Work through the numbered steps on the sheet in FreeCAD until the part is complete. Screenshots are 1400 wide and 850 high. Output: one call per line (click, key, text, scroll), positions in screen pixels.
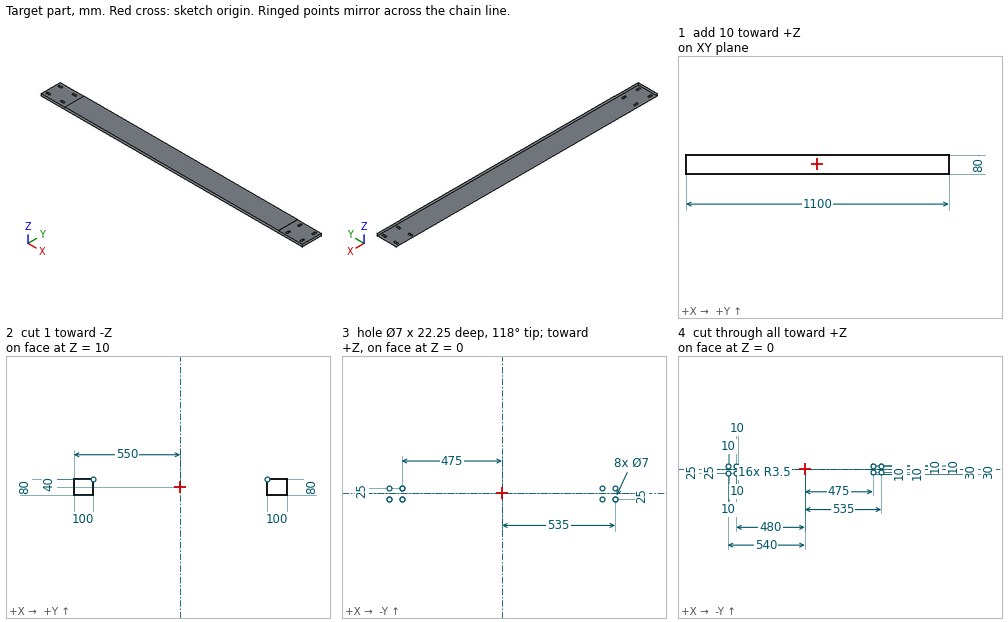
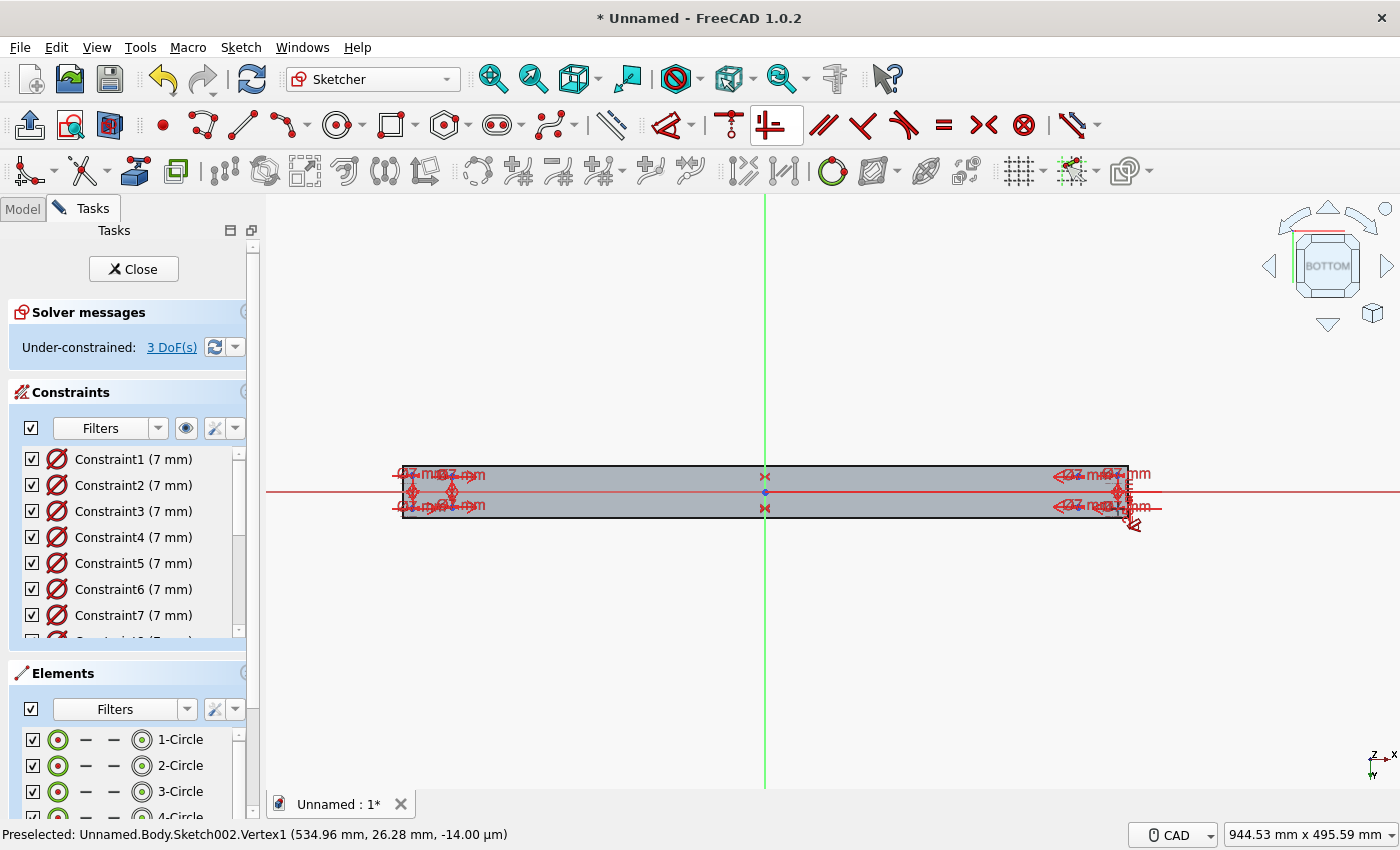
scroll(452, 477, up, 5)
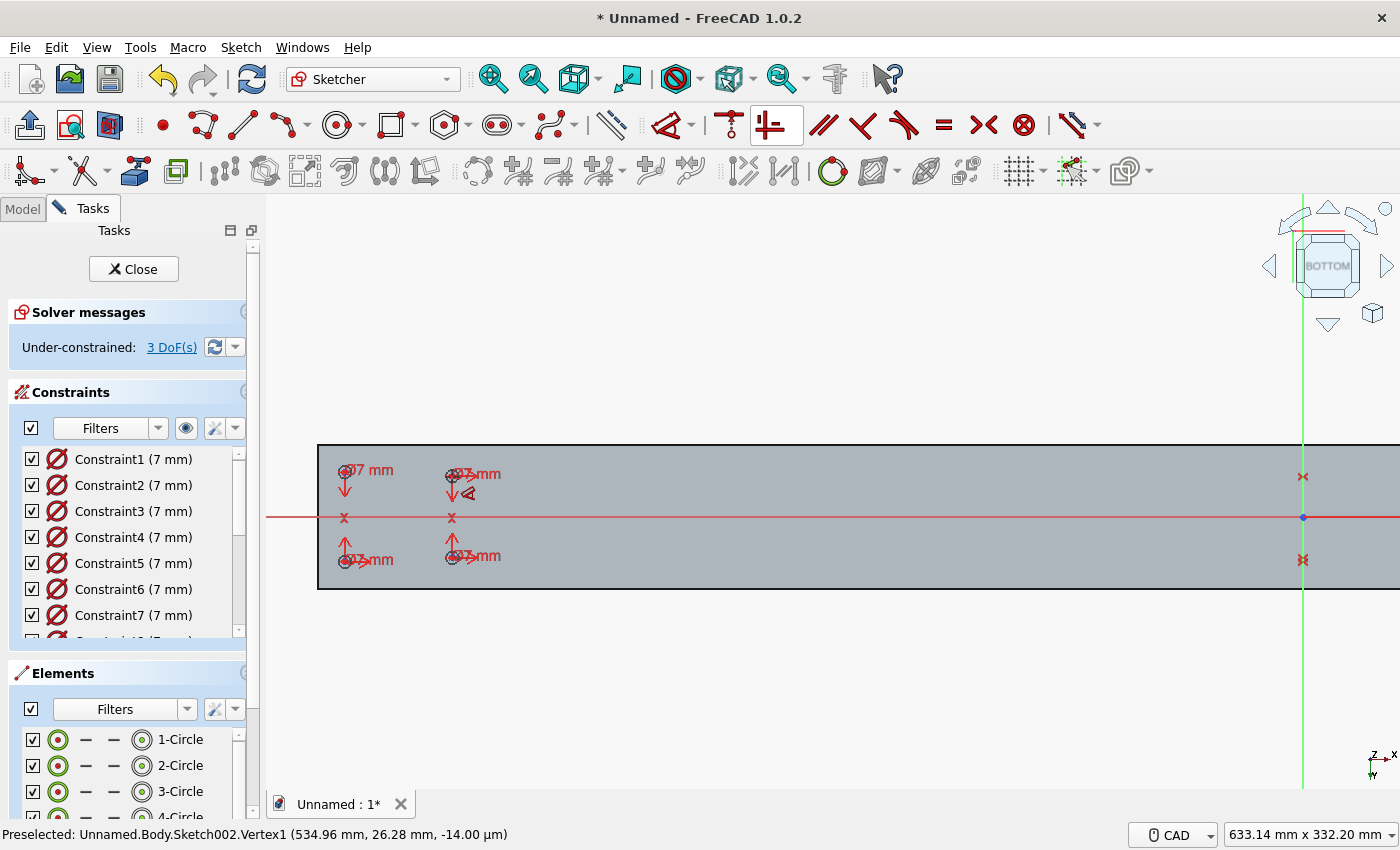
click(452, 476)
click(418, 497)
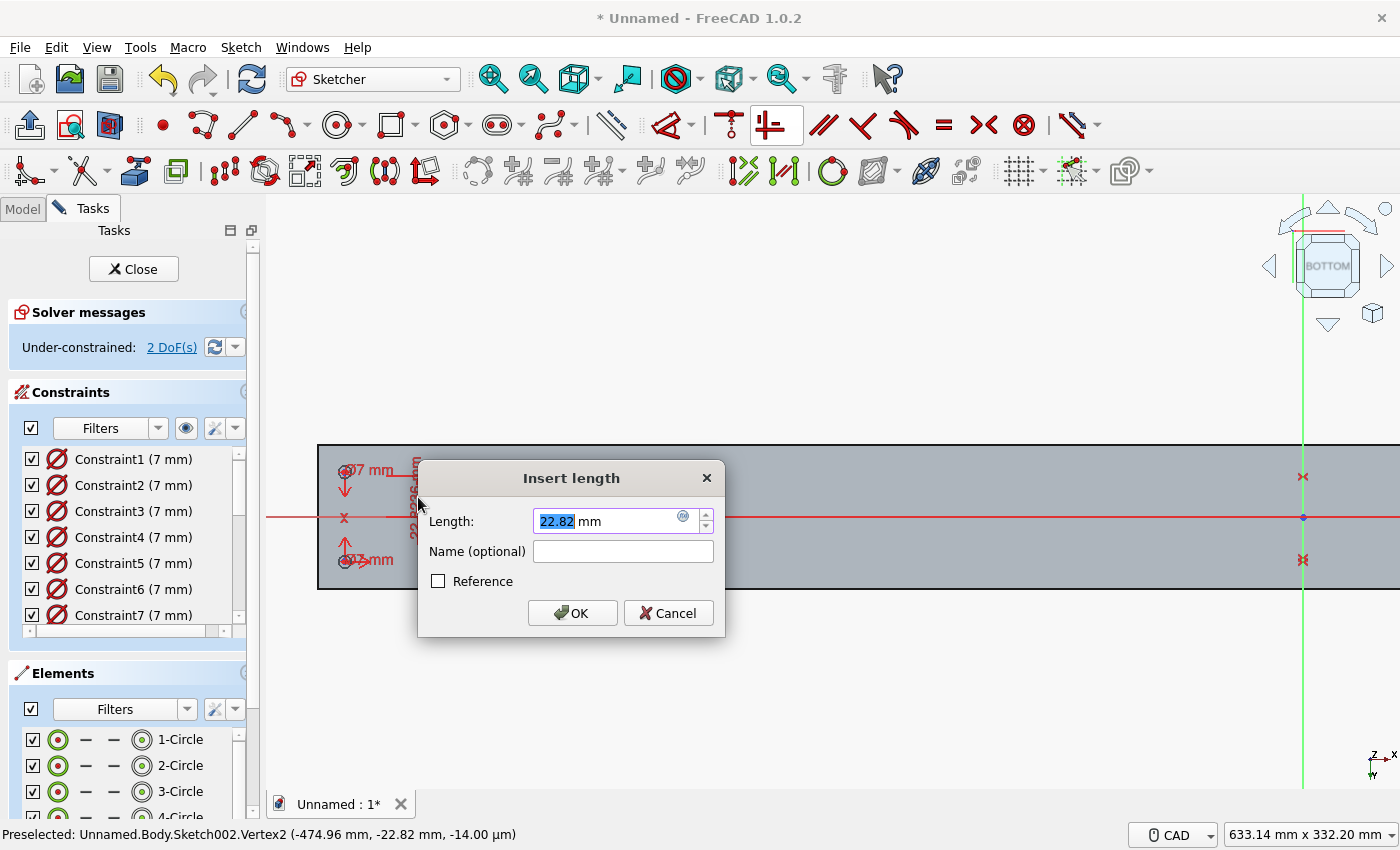
text(25)
key(Return)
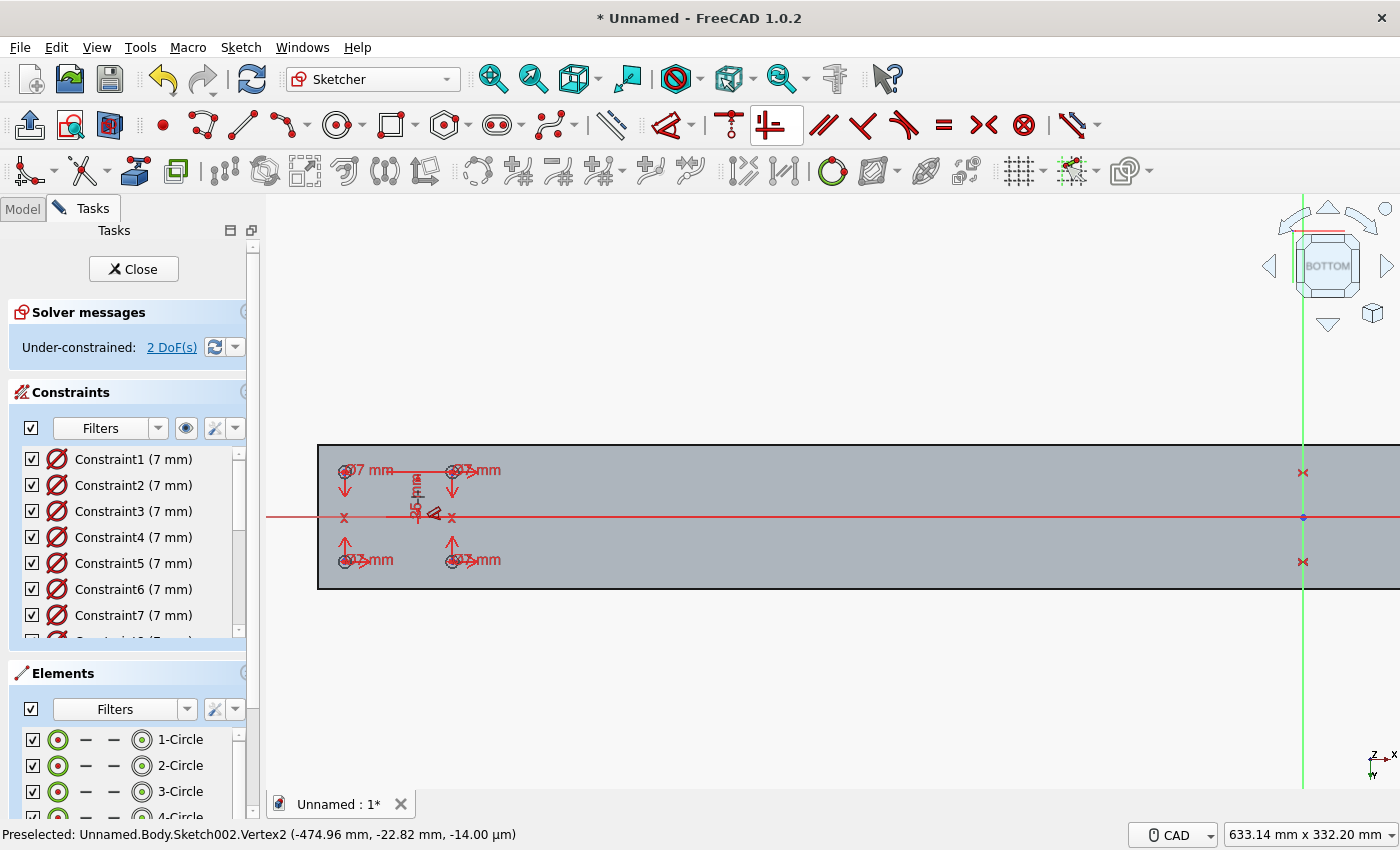
scroll(451, 477, down, 5)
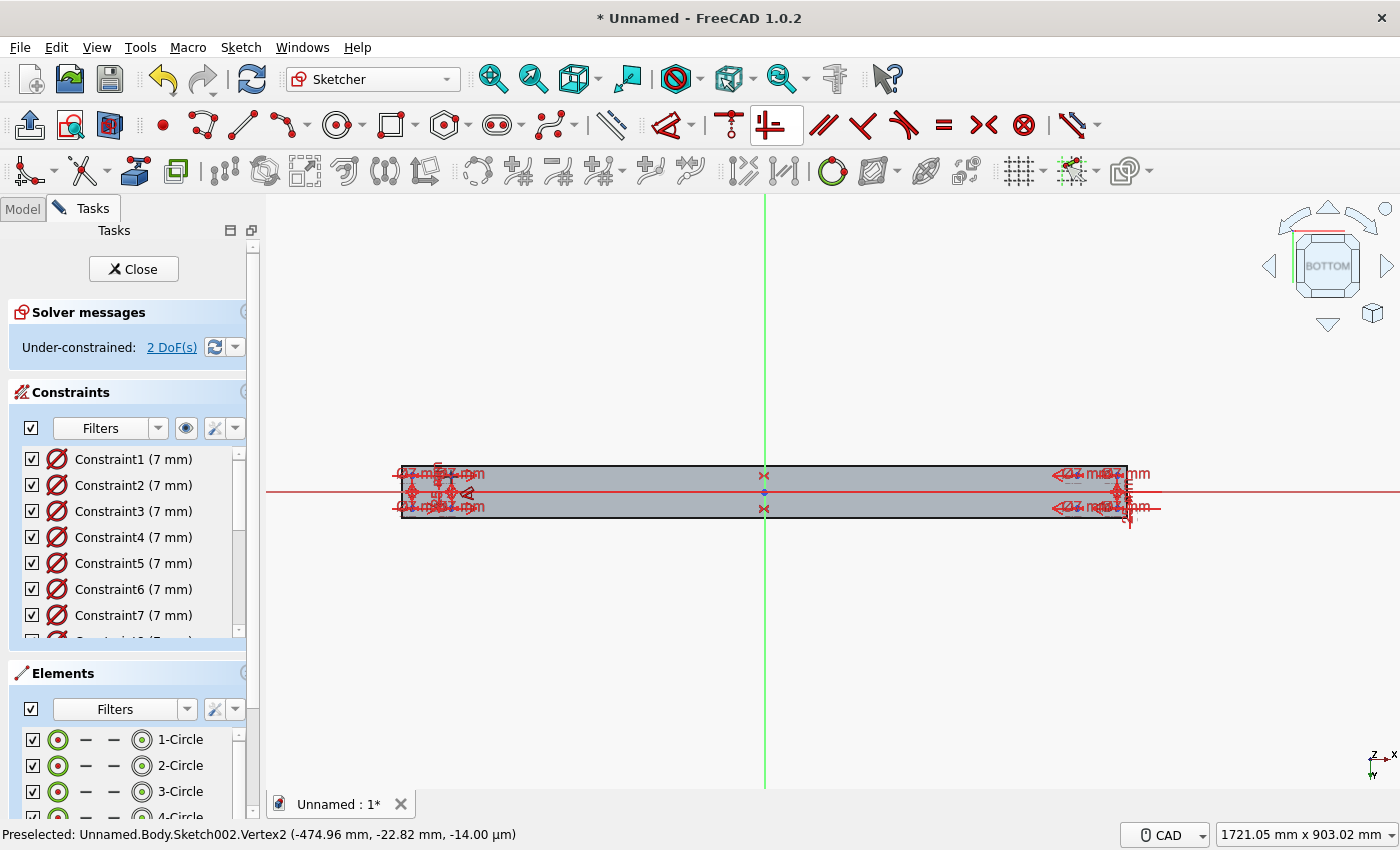
click(1117, 509)
click(941, 543)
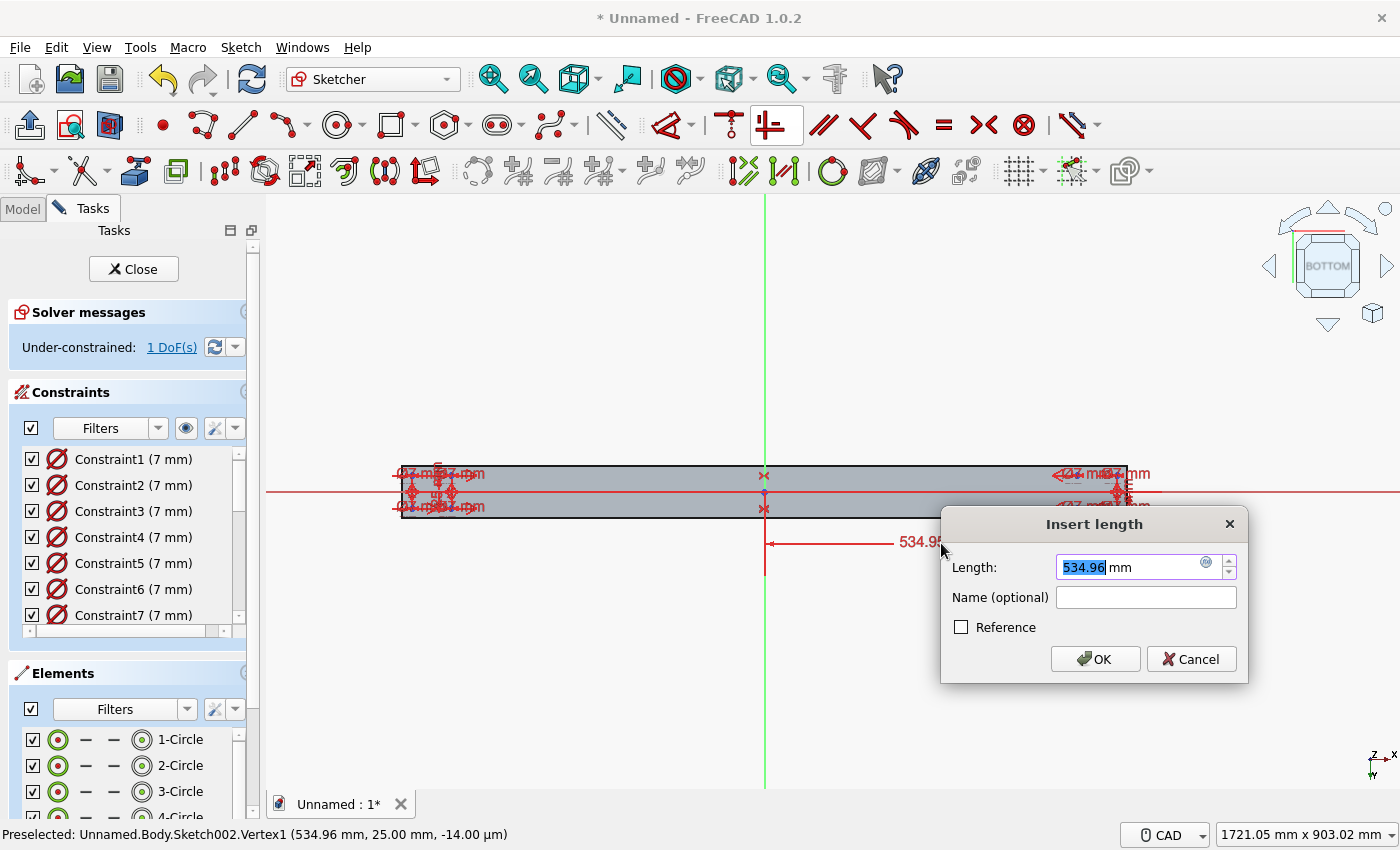
text(535)
key(Return)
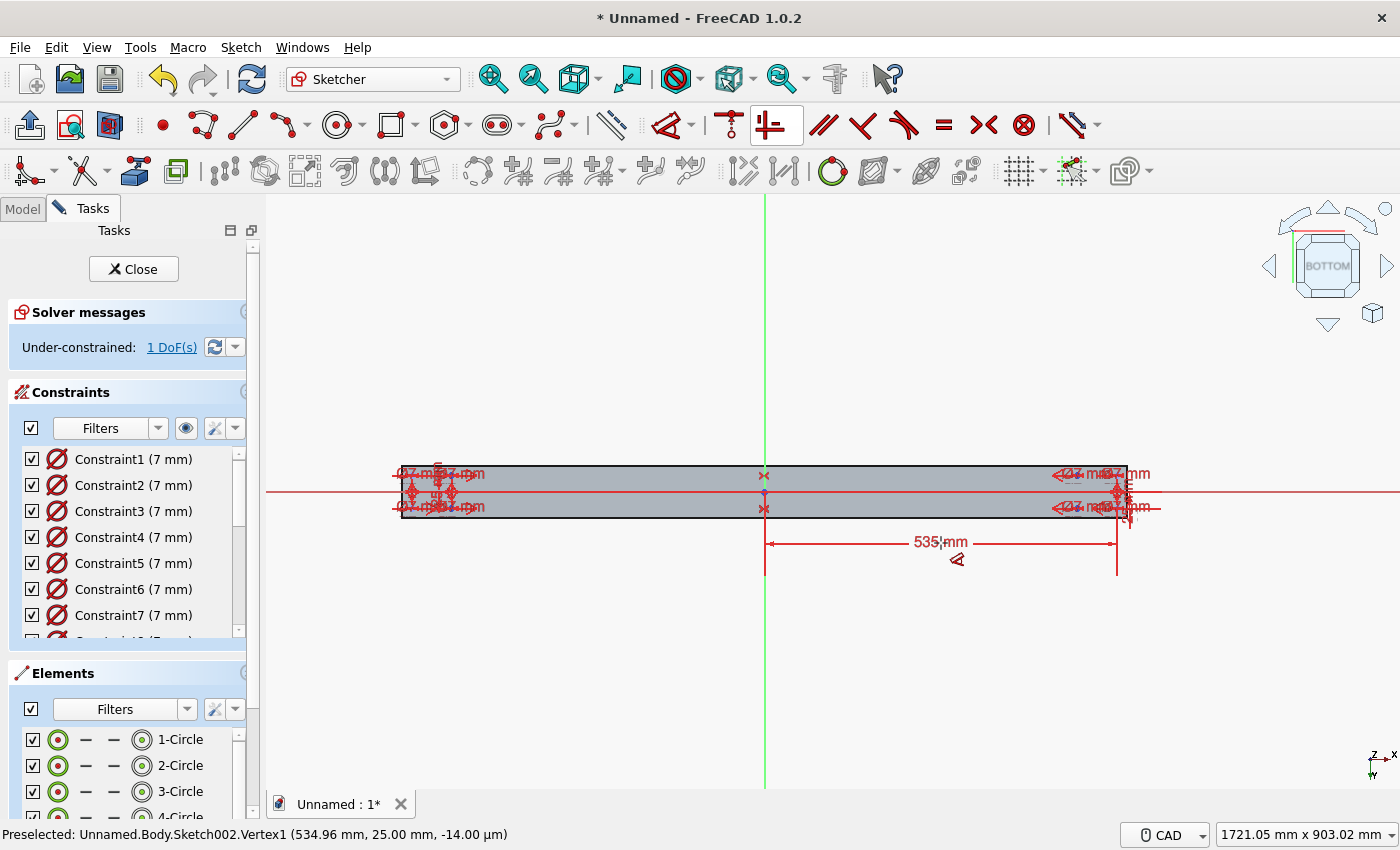
click(452, 476)
click(608, 442)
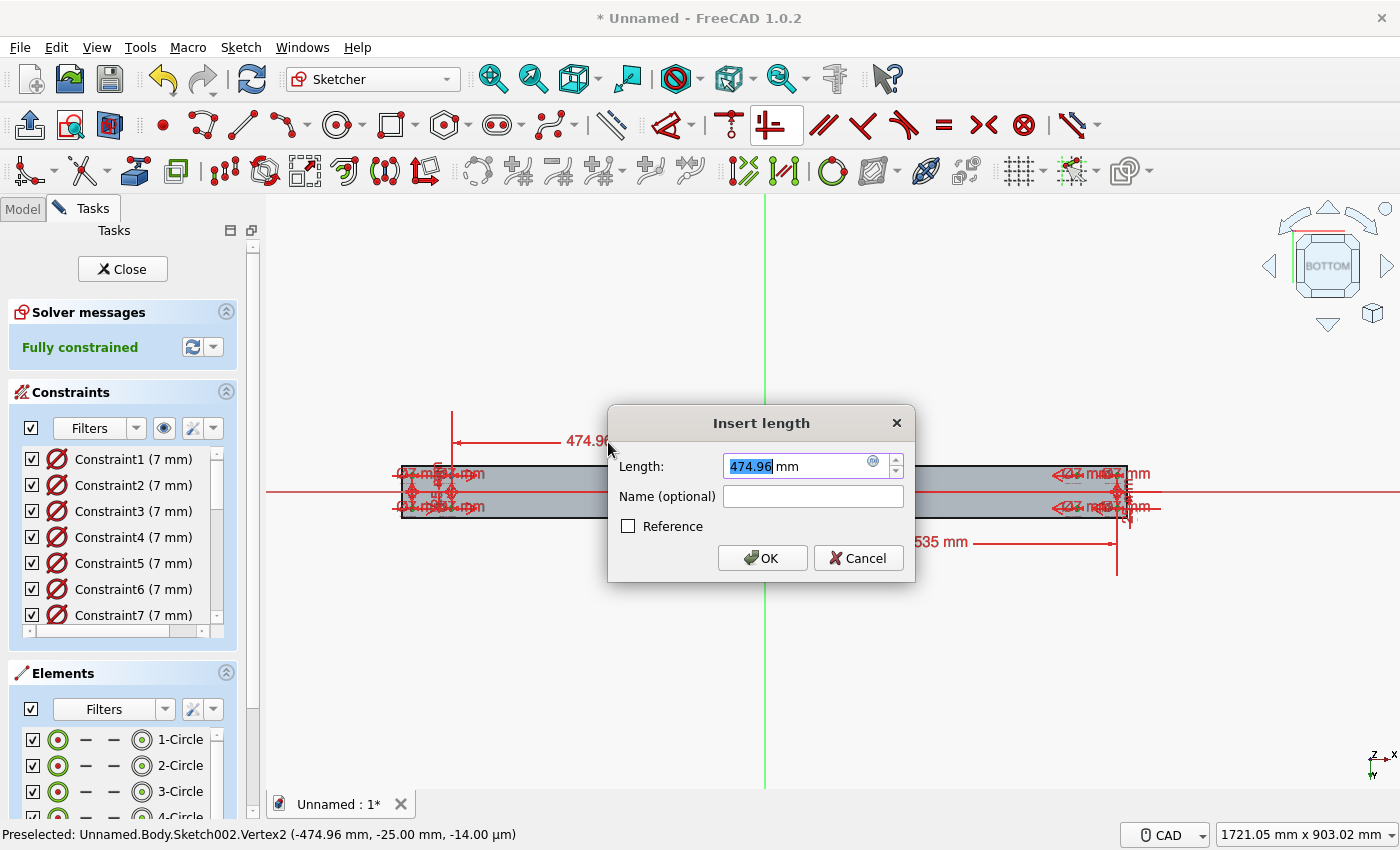
text(475)
key(Return)
key(Escape)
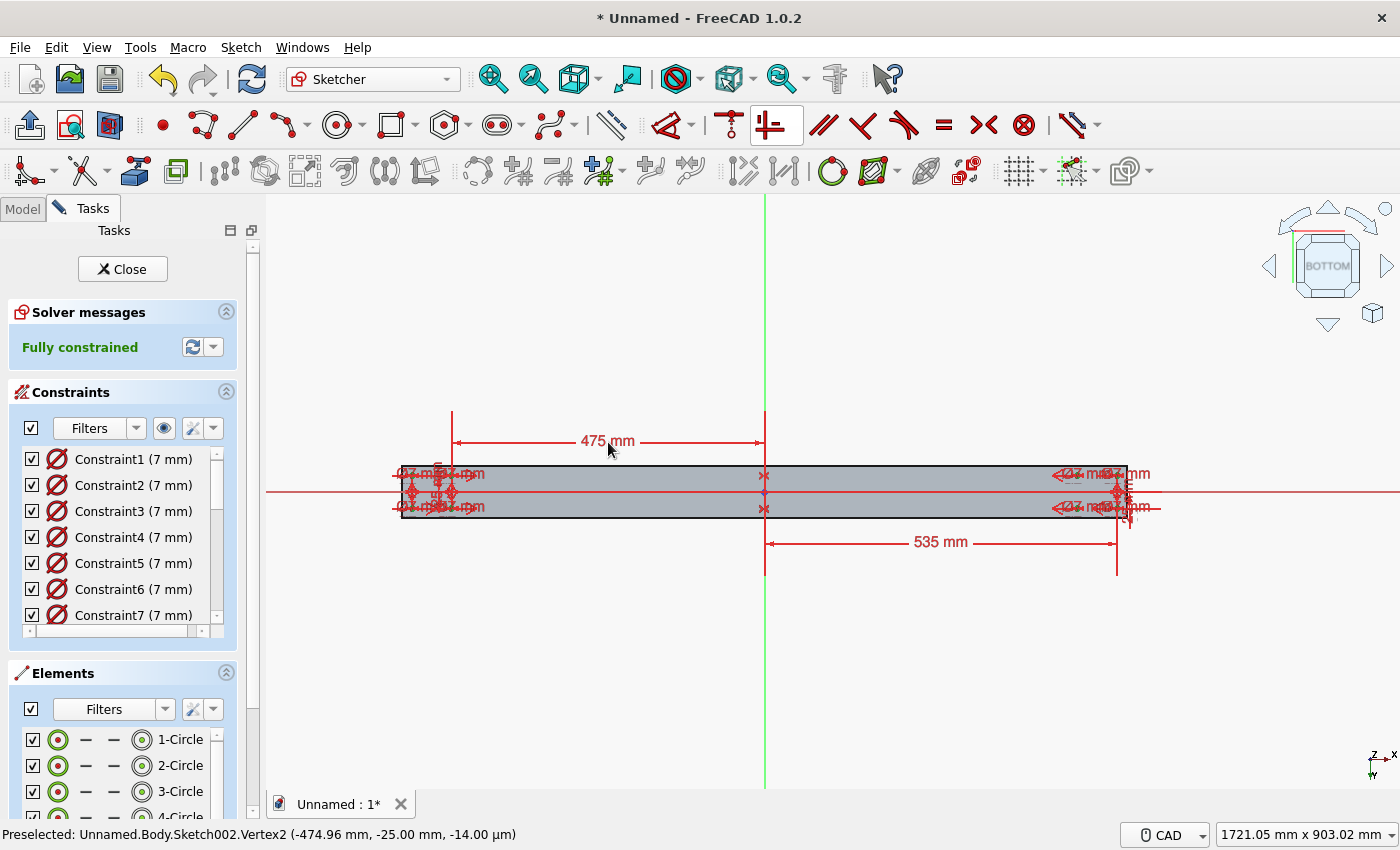
click(123, 269)